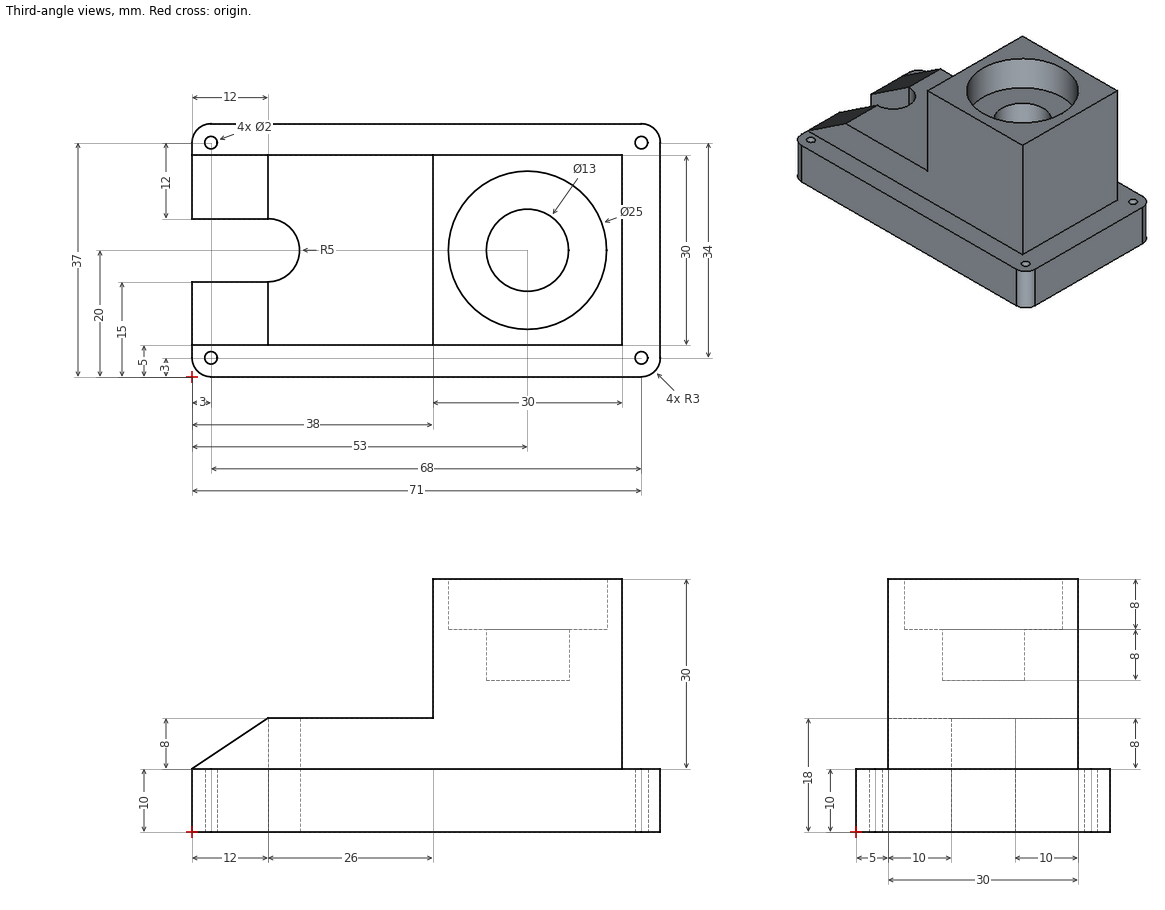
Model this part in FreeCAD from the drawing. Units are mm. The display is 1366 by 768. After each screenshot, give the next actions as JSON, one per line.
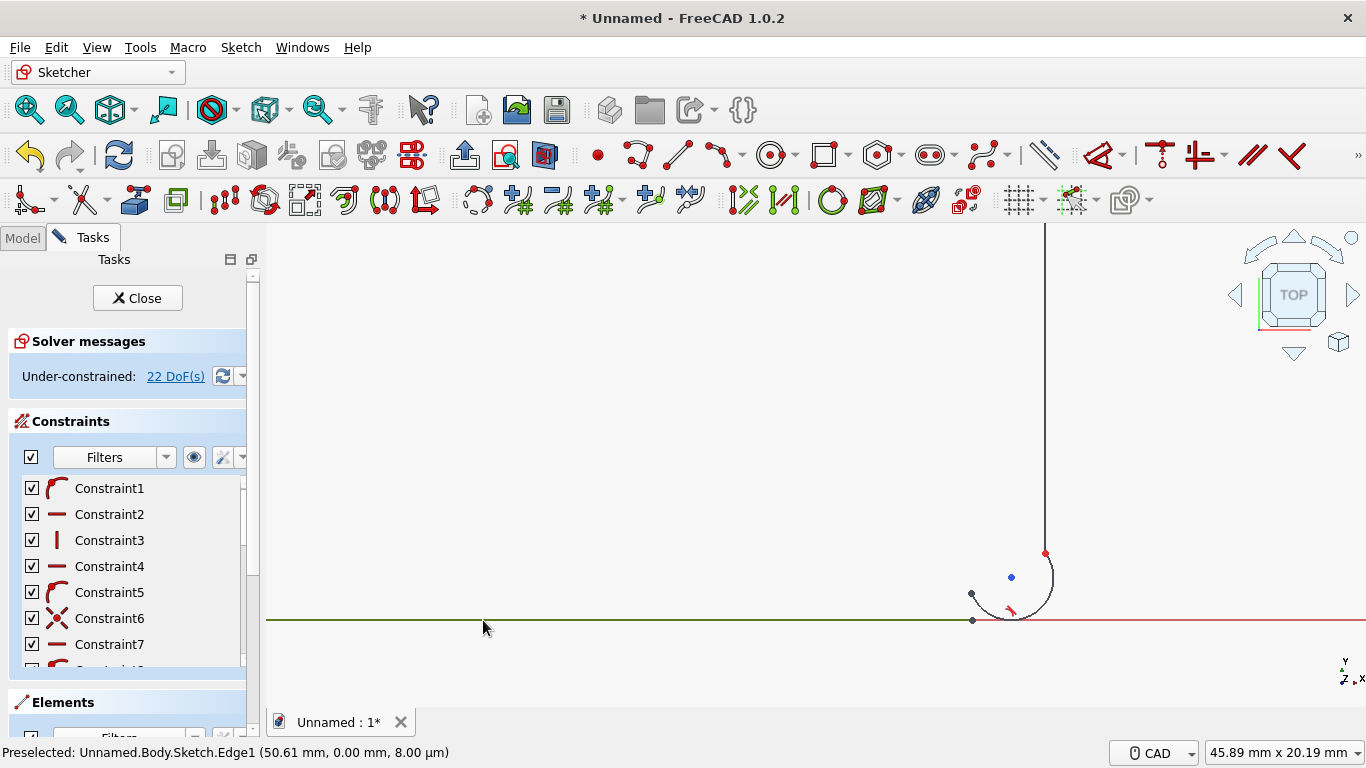
{"action": "scroll", "coordinate": [1002, 605], "scroll_direction": "down", "scroll_amount": 6}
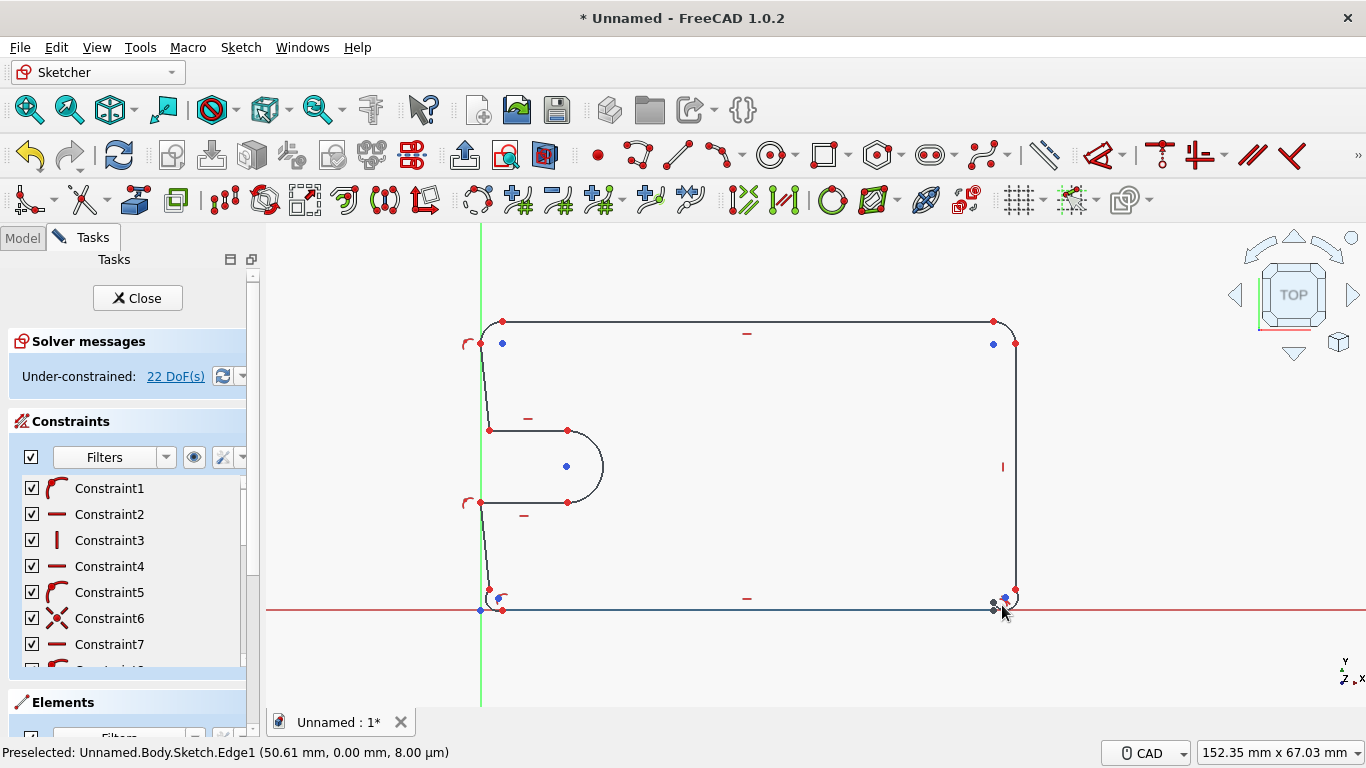
{"action": "scroll", "coordinate": [486, 599], "scroll_direction": "up", "scroll_amount": 5}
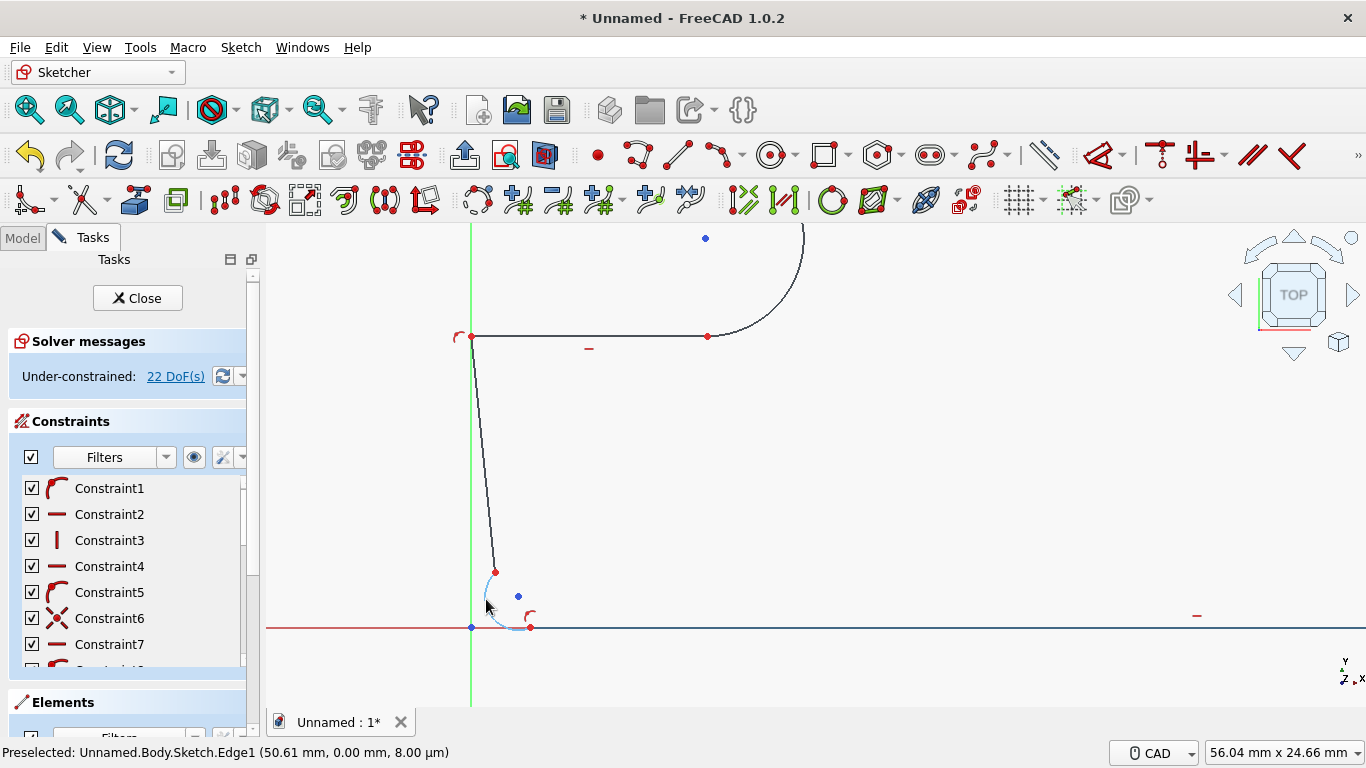
{"action": "left_click", "coordinate": [485, 598]}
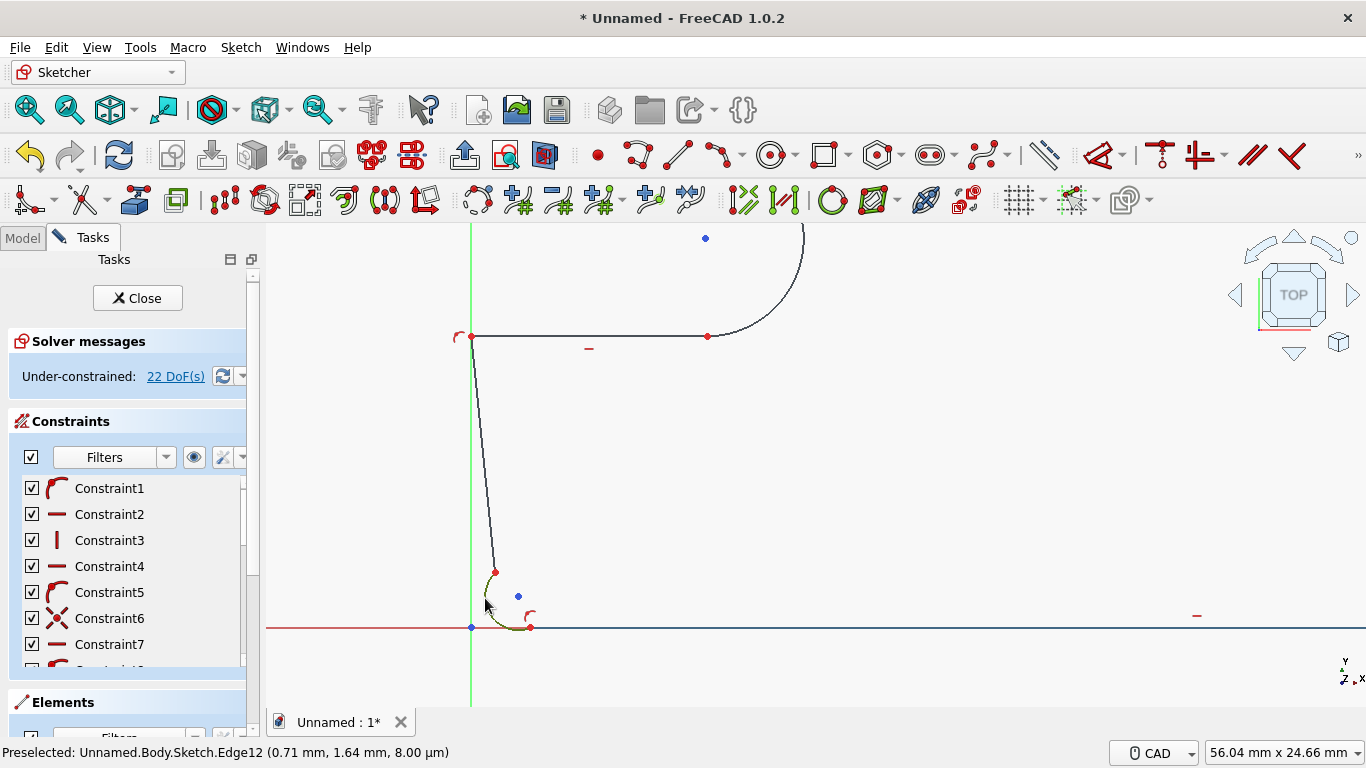
{"action": "key", "text": "t"}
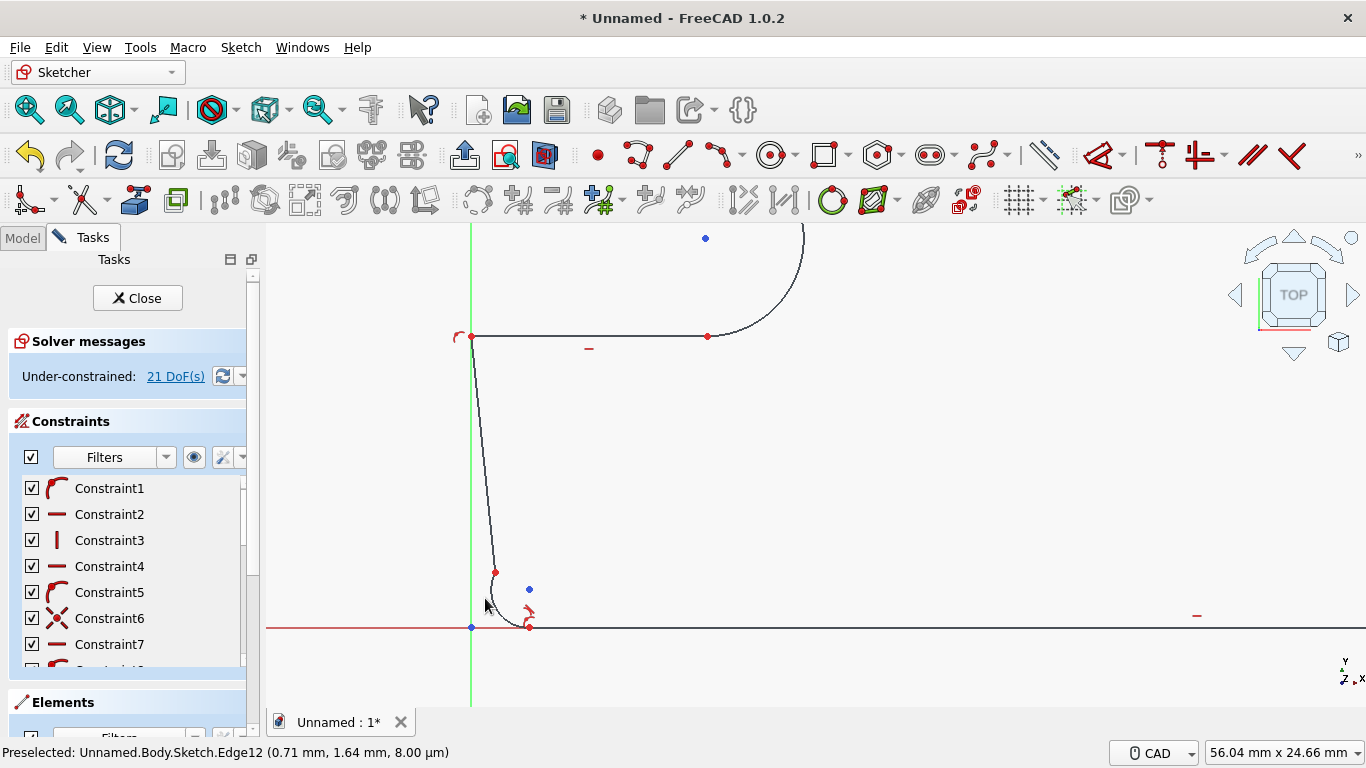
{"action": "scroll", "coordinate": [486, 599], "scroll_direction": "down", "scroll_amount": 5}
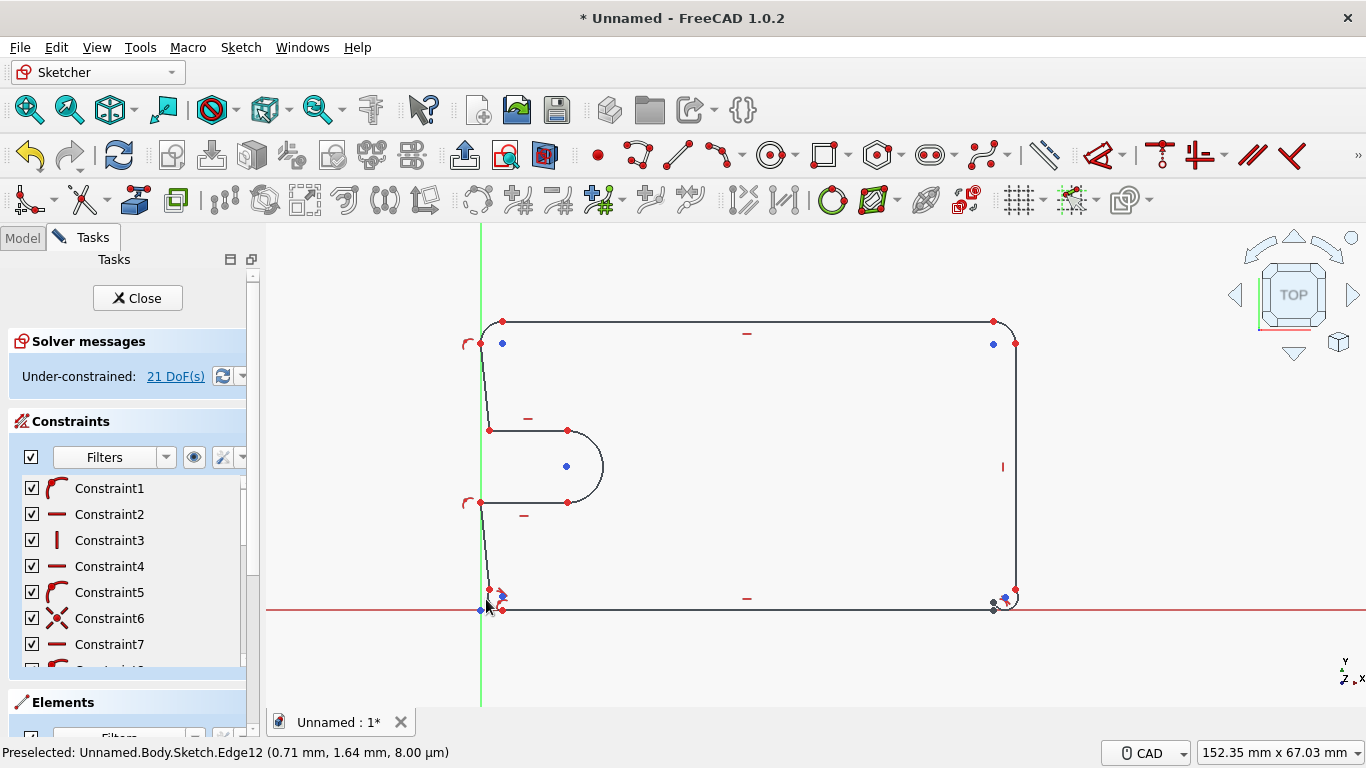
{"action": "left_click", "coordinate": [1016, 516]}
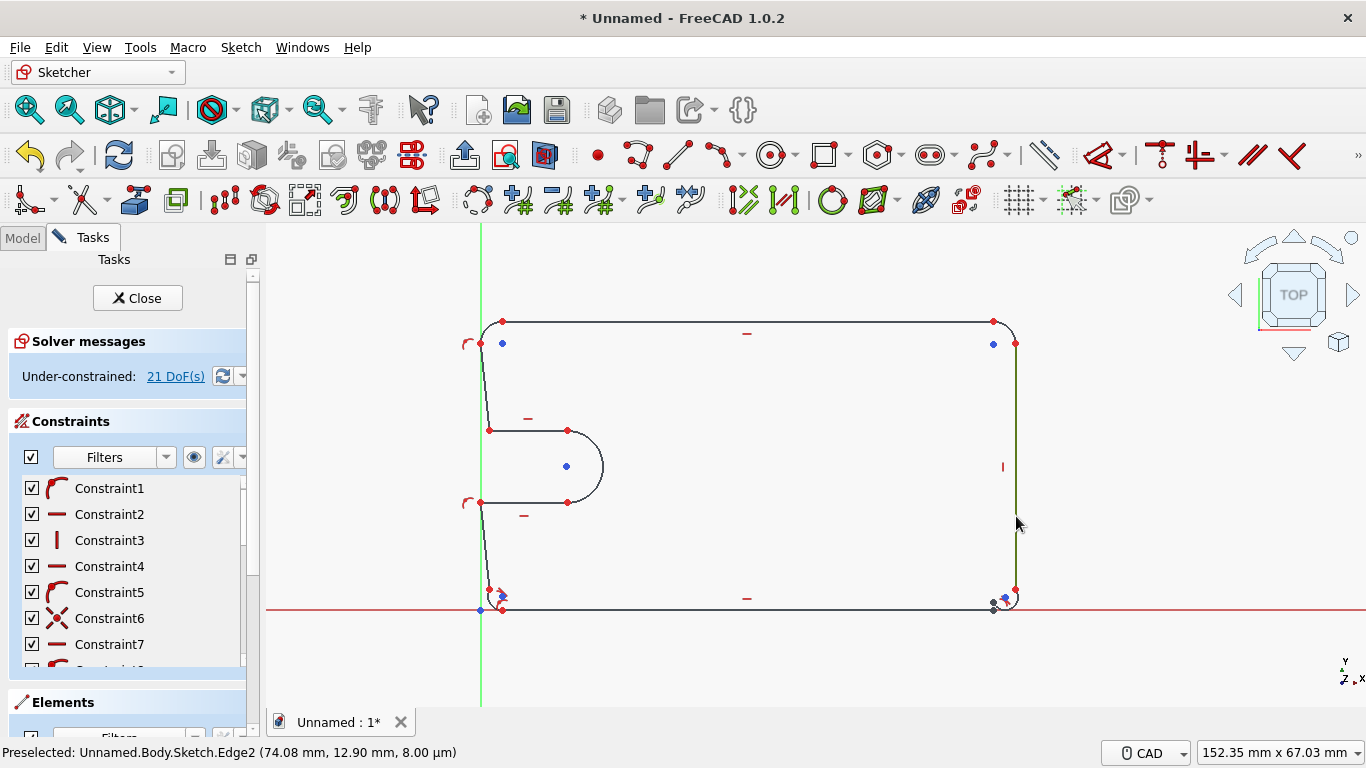
{"action": "scroll", "coordinate": [1003, 610], "scroll_direction": "up", "scroll_amount": 2}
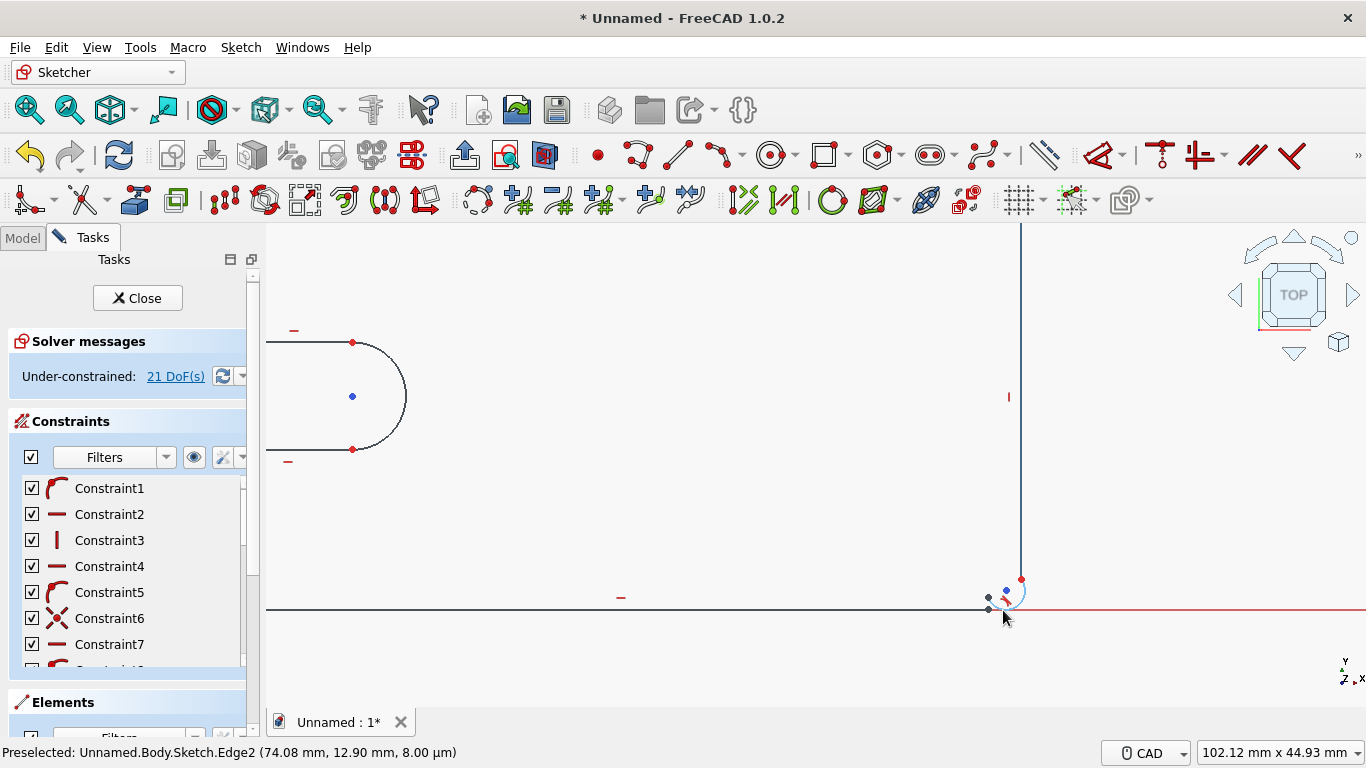
{"action": "left_click", "coordinate": [1003, 609]}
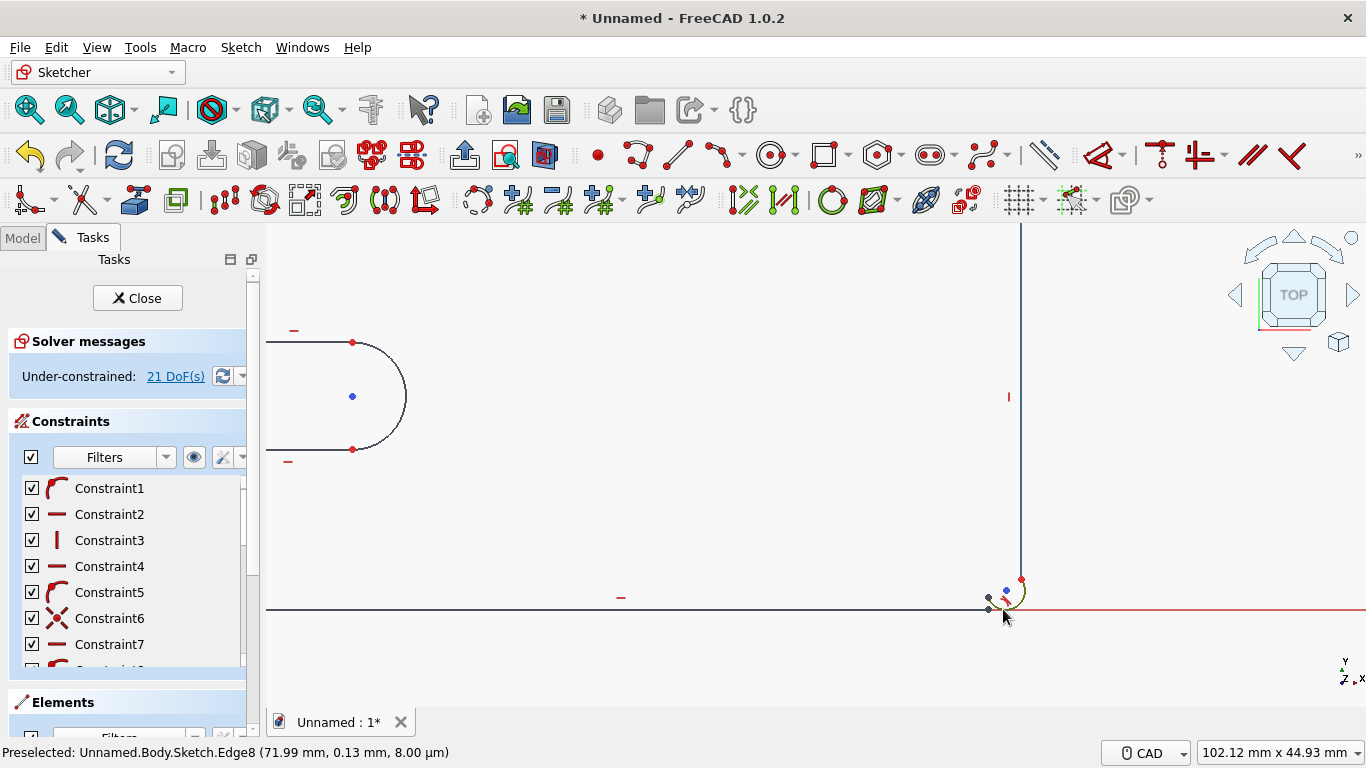
{"action": "key", "text": "t"}